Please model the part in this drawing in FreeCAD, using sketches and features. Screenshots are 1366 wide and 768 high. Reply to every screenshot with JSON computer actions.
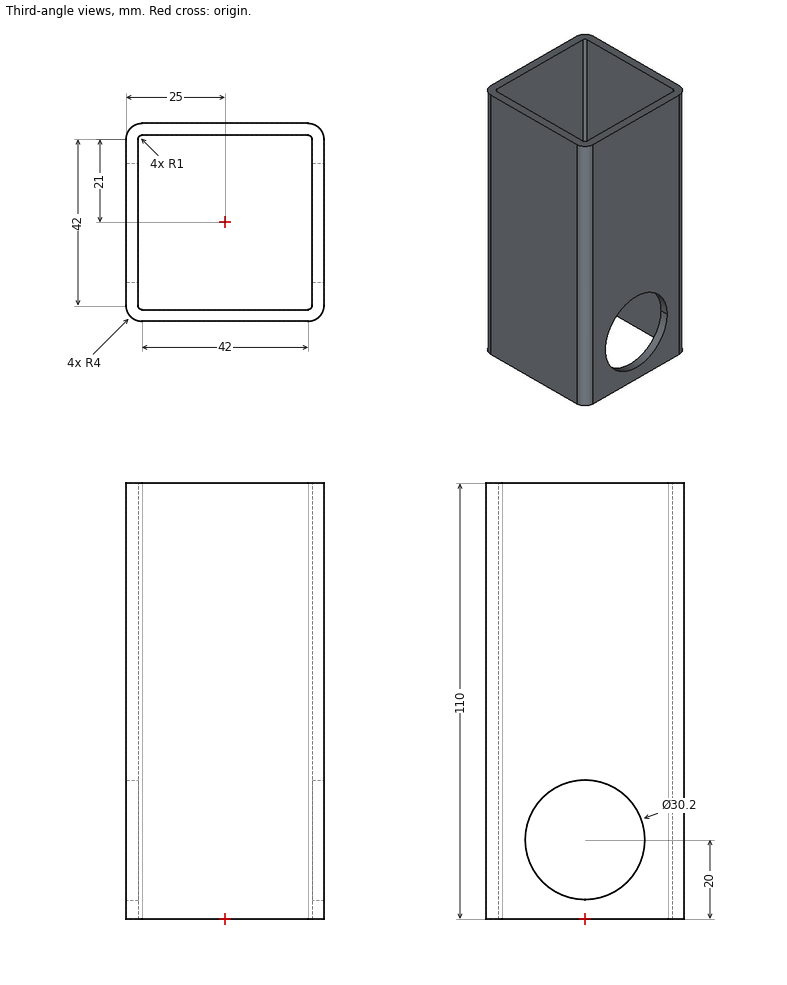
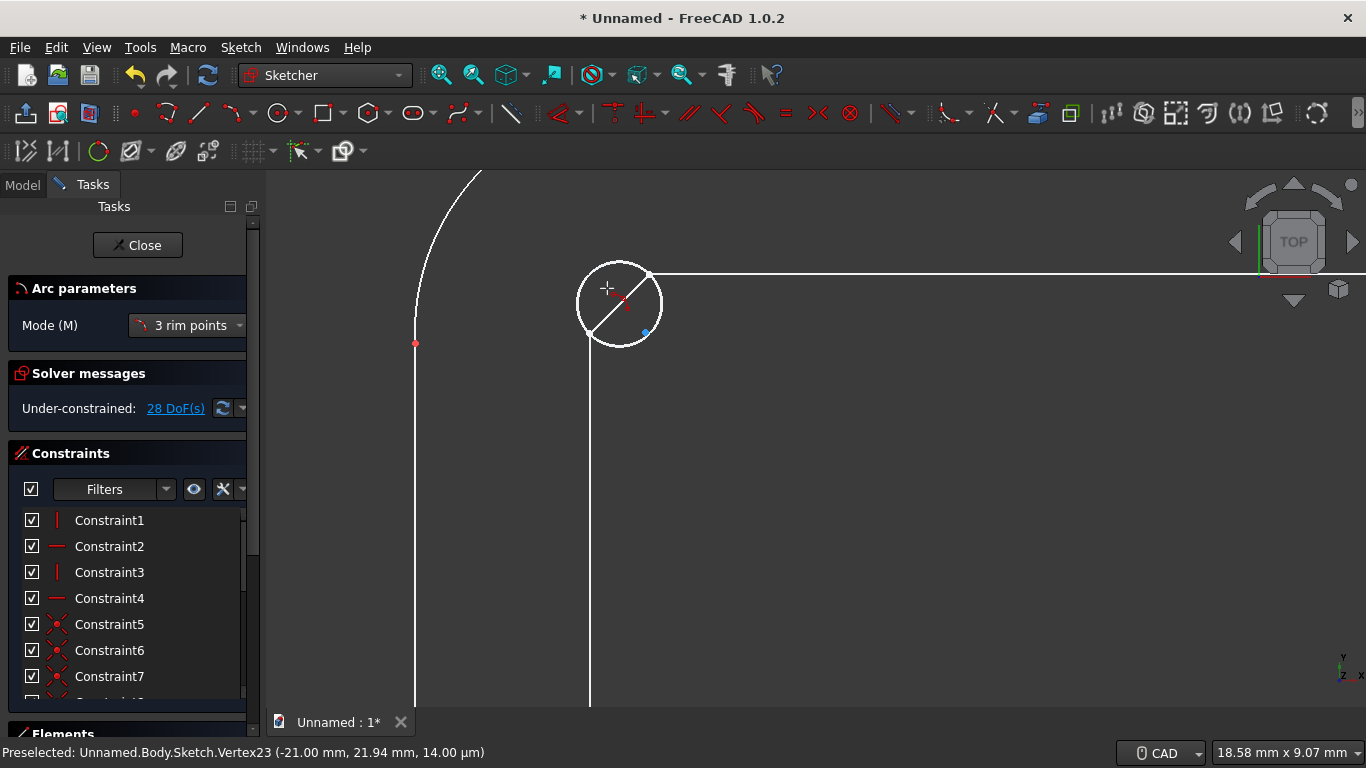
{"action": "left_click", "coordinate": [607, 288]}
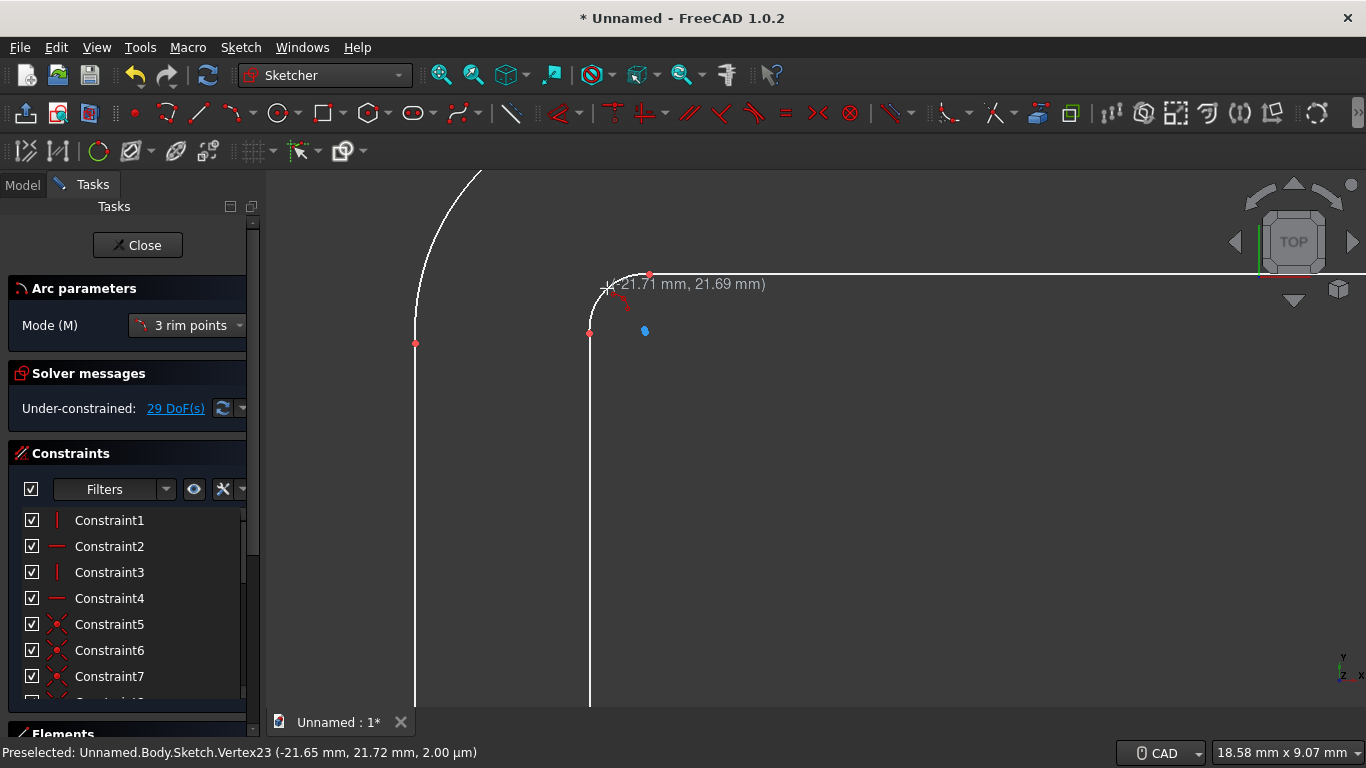
{"action": "scroll", "coordinate": [605, 297], "scroll_direction": "down", "scroll_amount": 11}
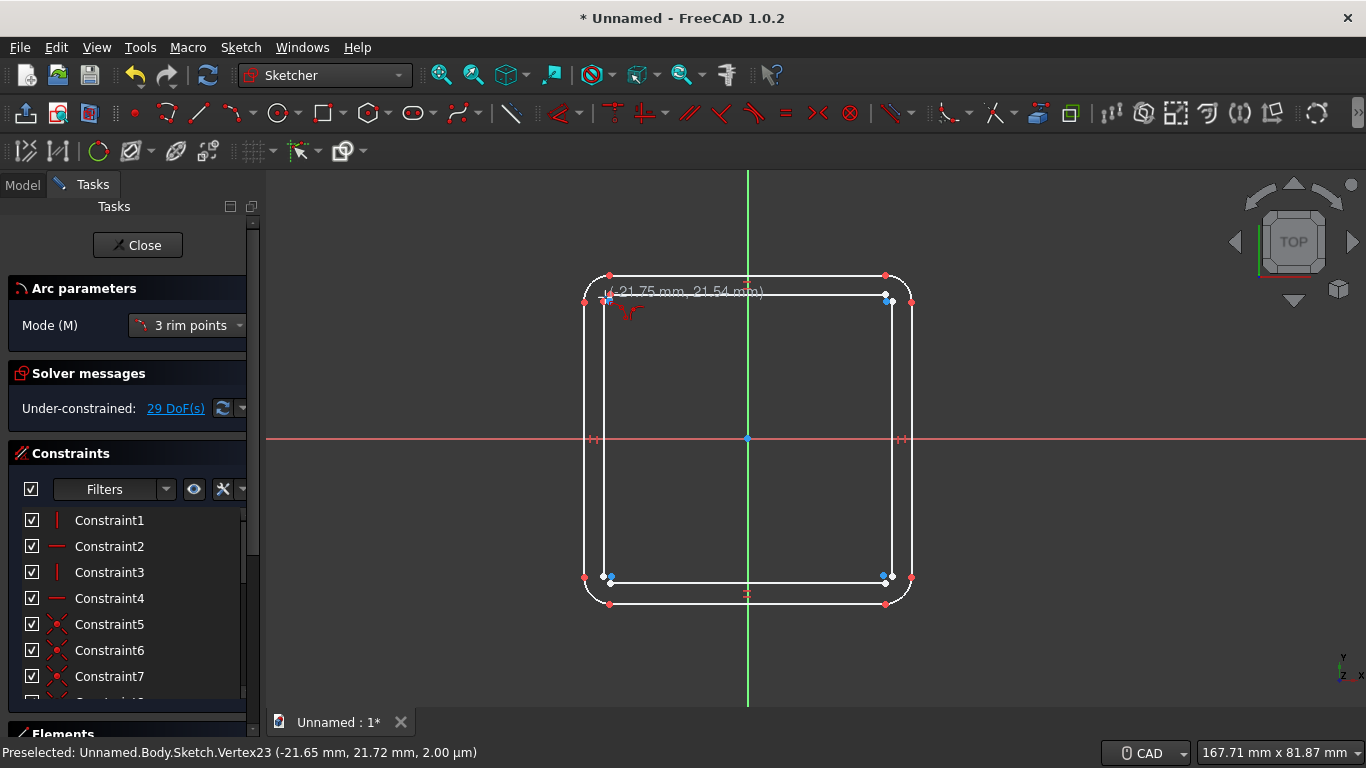
{"action": "scroll", "coordinate": [886, 294], "scroll_direction": "up", "scroll_amount": 5}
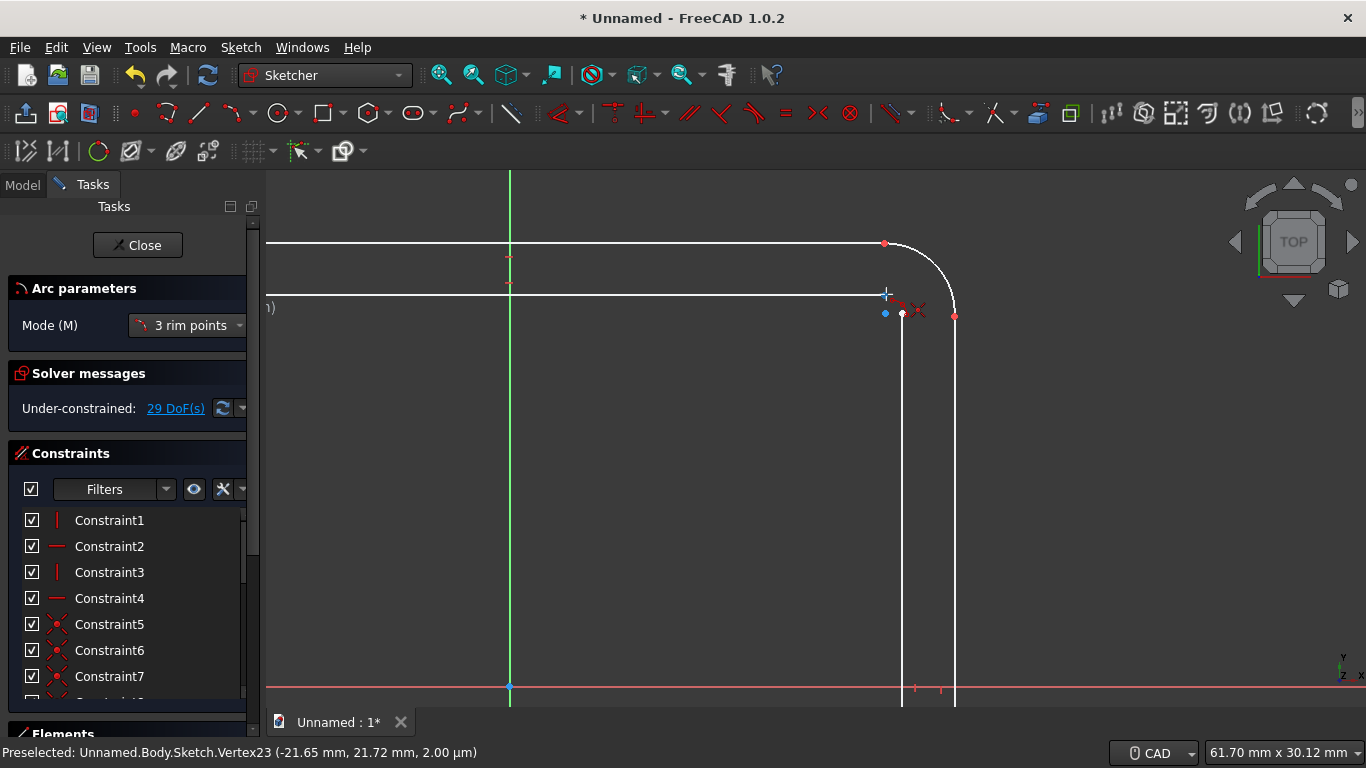
{"action": "left_click", "coordinate": [884, 295]}
{"action": "left_click", "coordinate": [902, 313]}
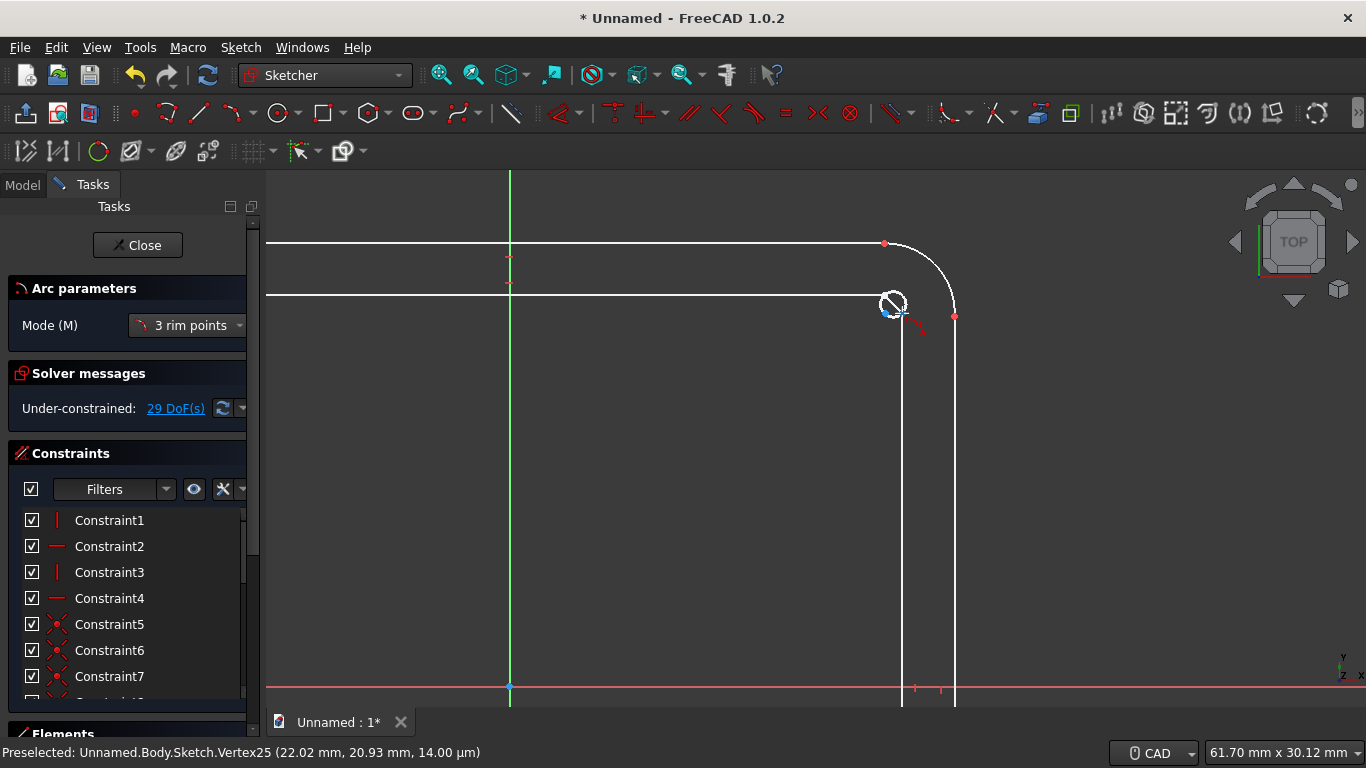
{"action": "scroll", "coordinate": [897, 300], "scroll_direction": "up", "scroll_amount": 6}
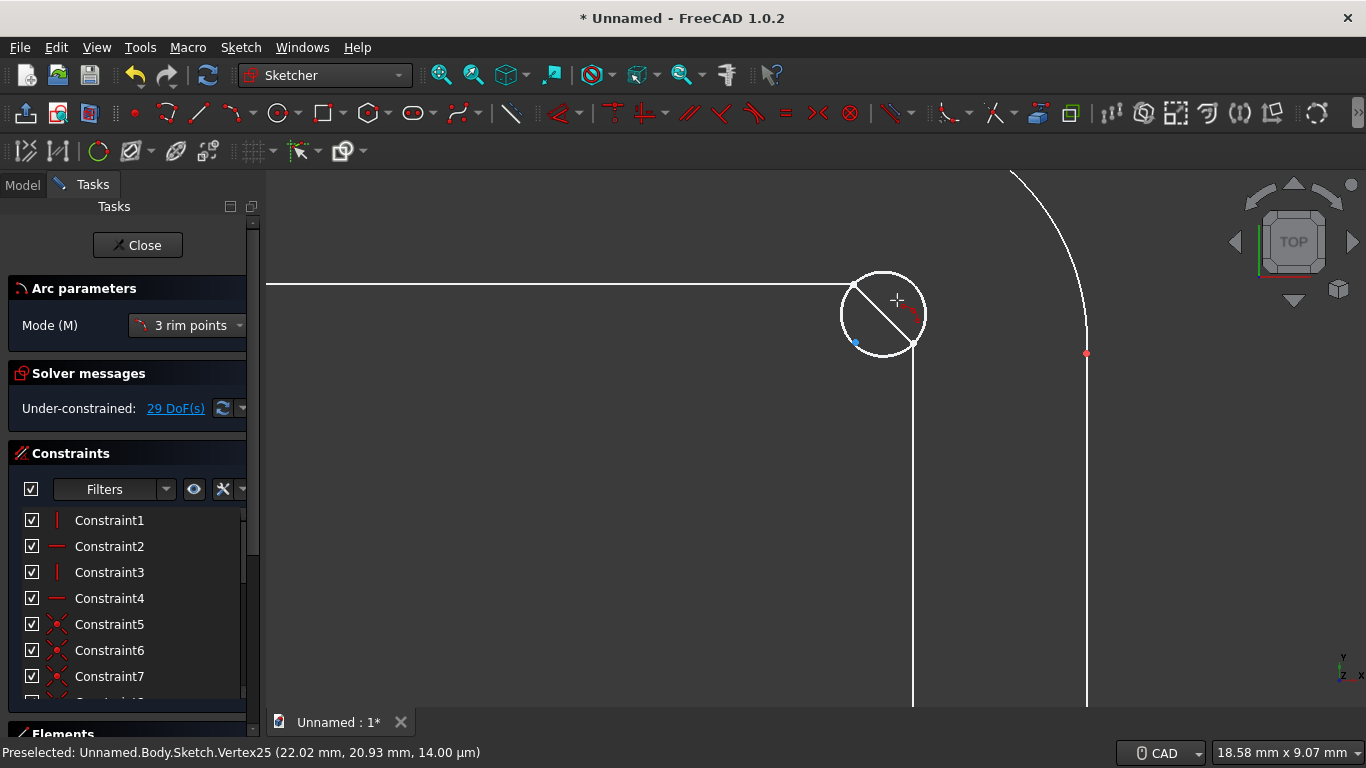
{"action": "left_click", "coordinate": [895, 298]}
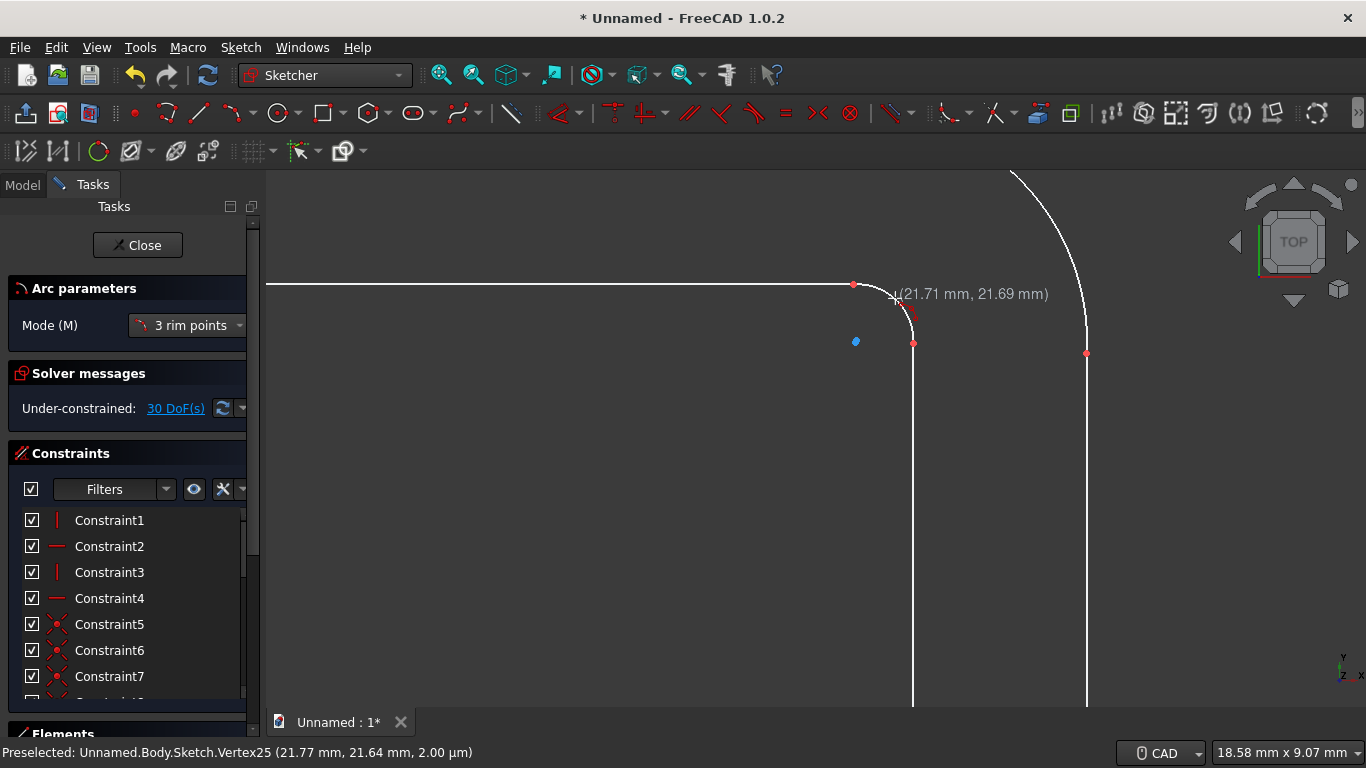
{"action": "scroll", "coordinate": [889, 296], "scroll_direction": "down", "scroll_amount": 11}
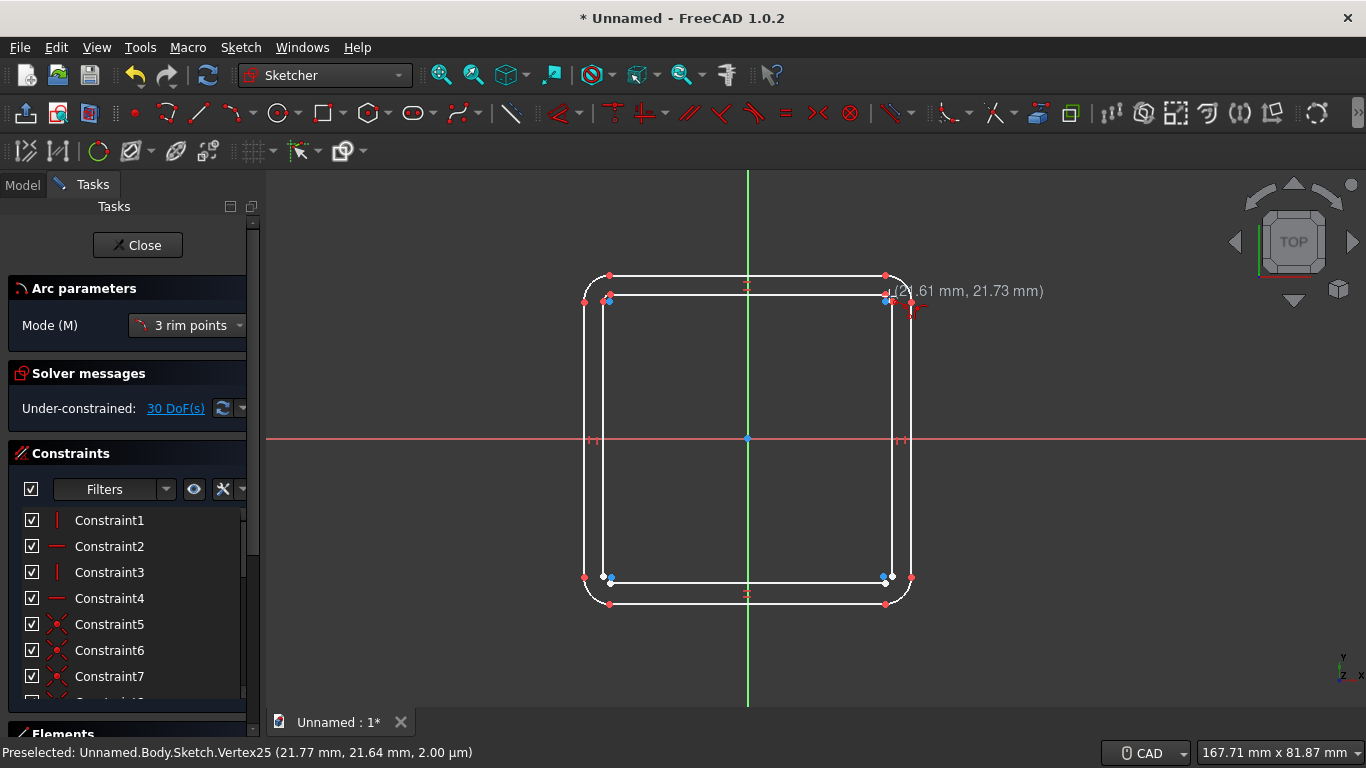
{"action": "scroll", "coordinate": [892, 577], "scroll_direction": "up", "scroll_amount": 5}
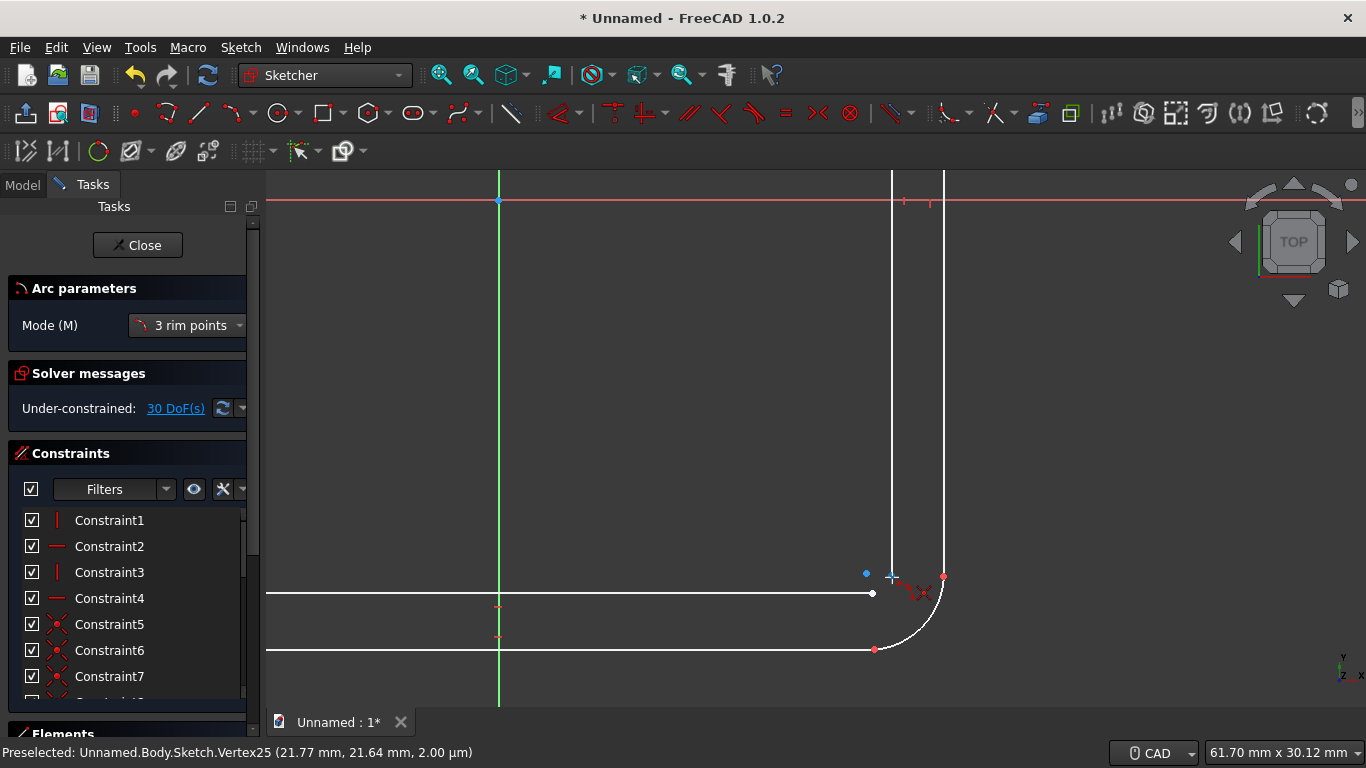
{"action": "left_click", "coordinate": [892, 575]}
{"action": "left_click", "coordinate": [873, 593]}